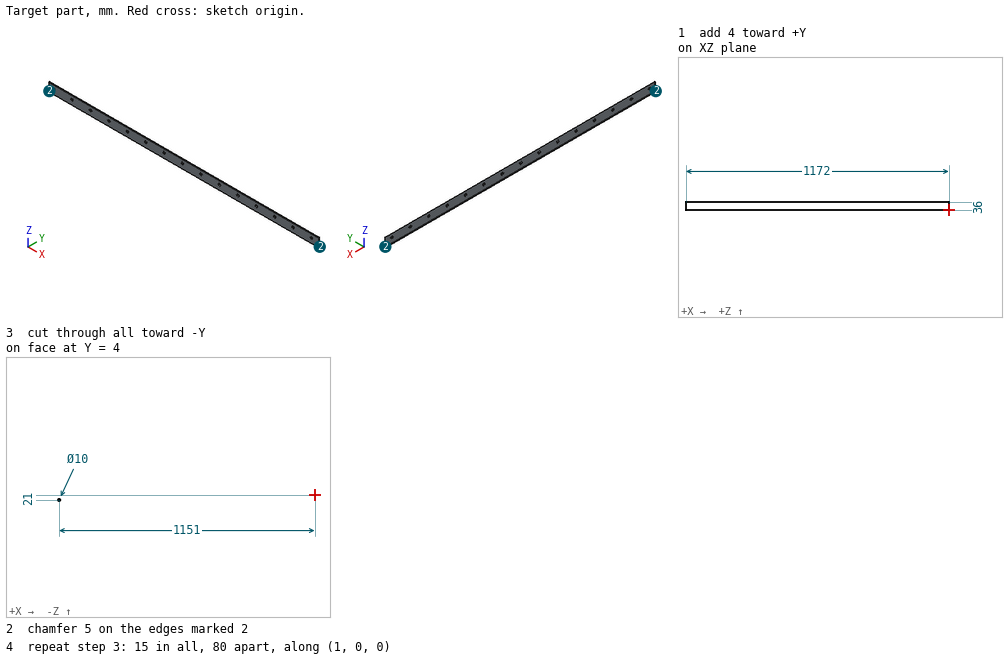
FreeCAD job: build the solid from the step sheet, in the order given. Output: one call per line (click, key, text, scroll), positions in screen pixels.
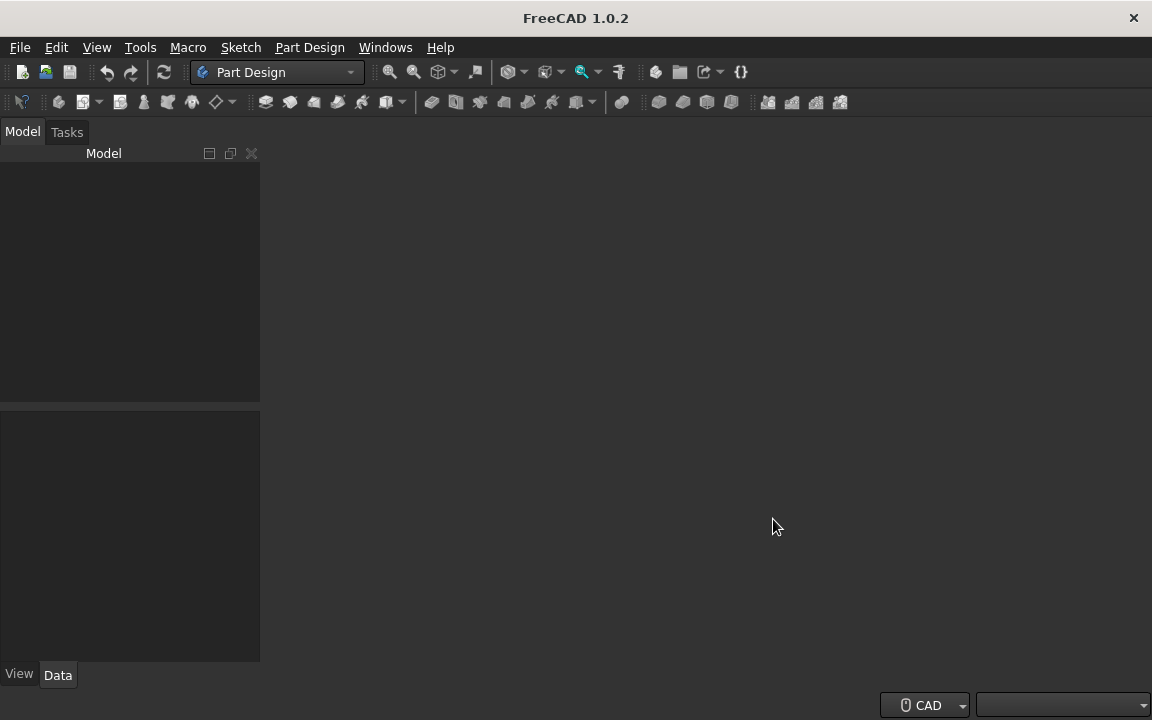
click(22, 72)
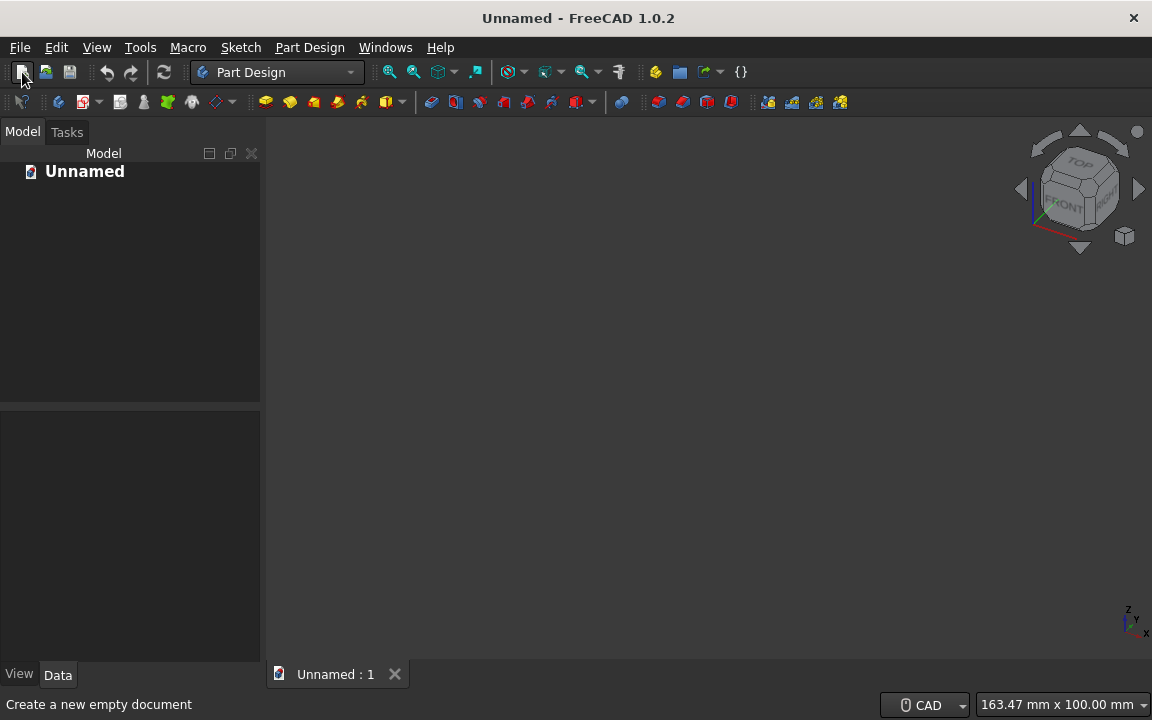
click(84, 102)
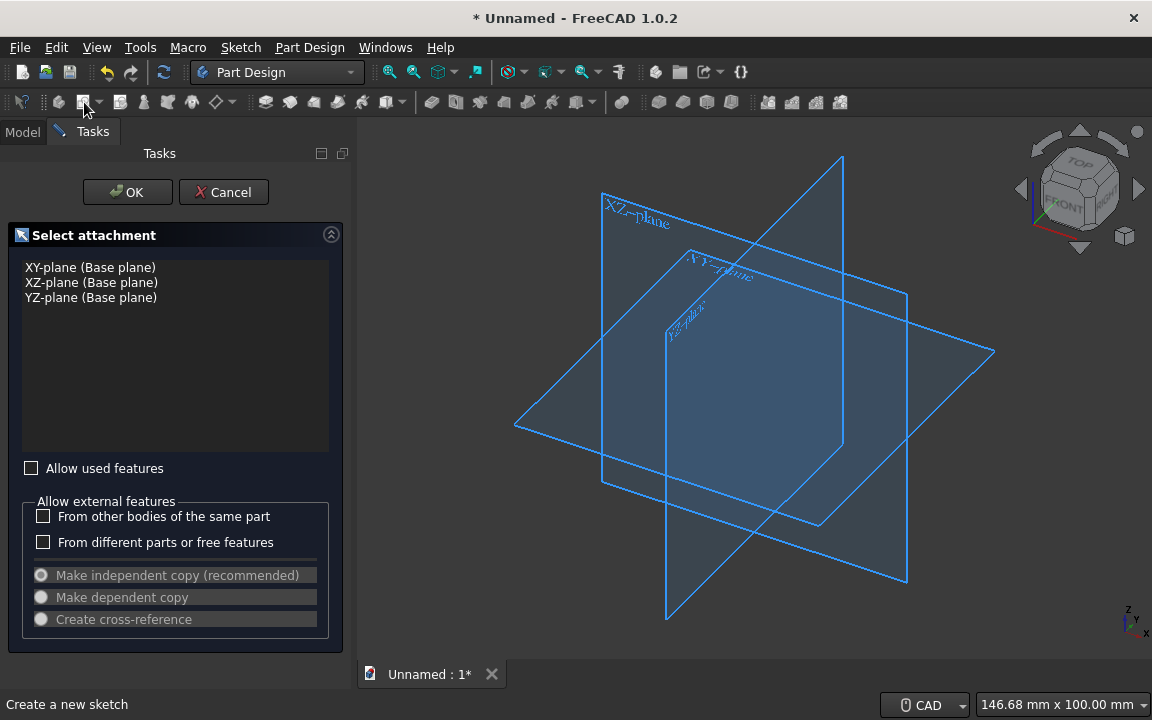
click(82, 282)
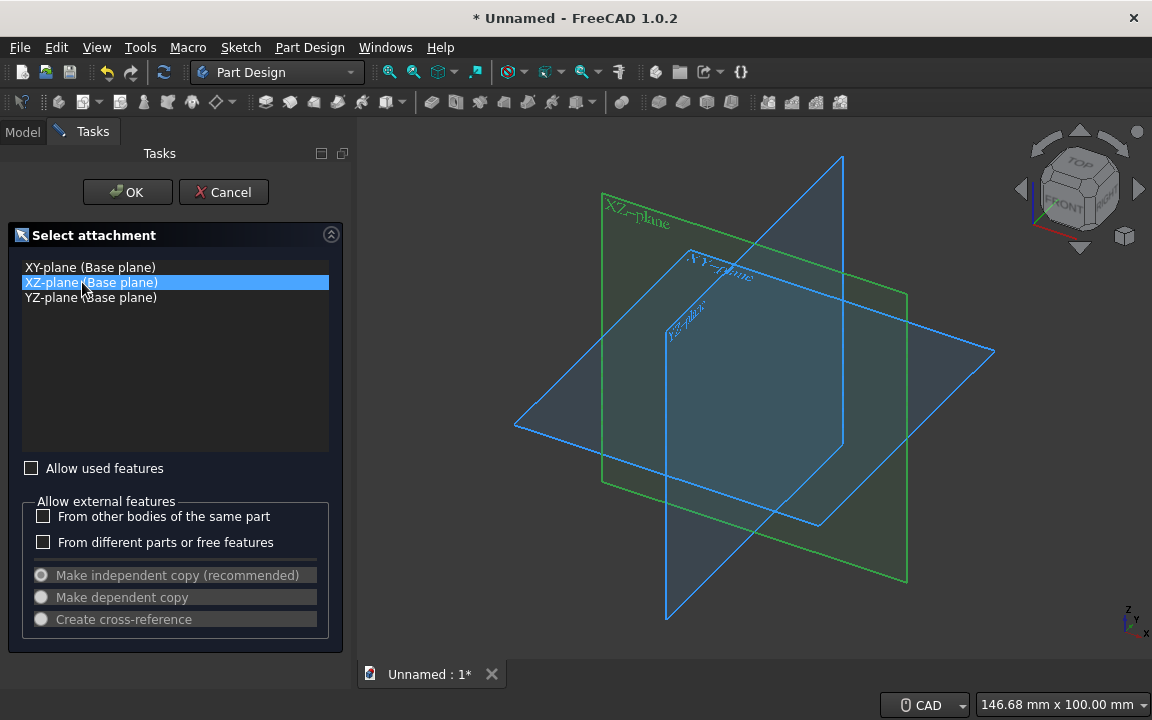
click(128, 192)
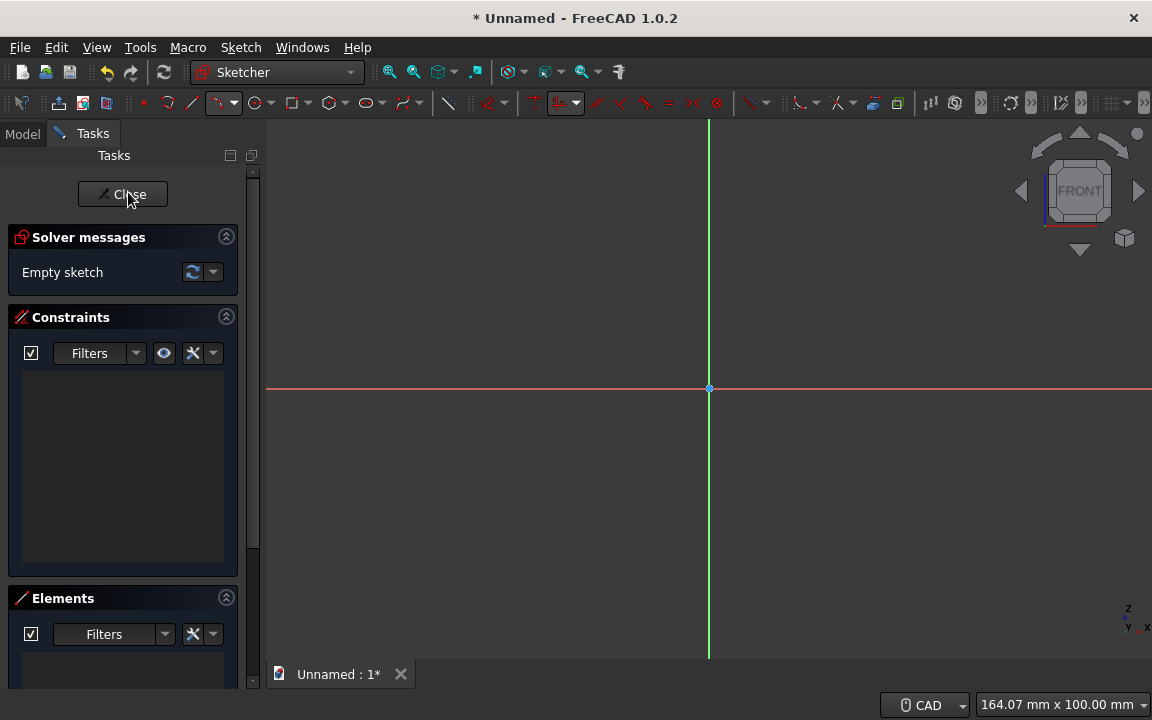
scroll(889, 397, down, 13)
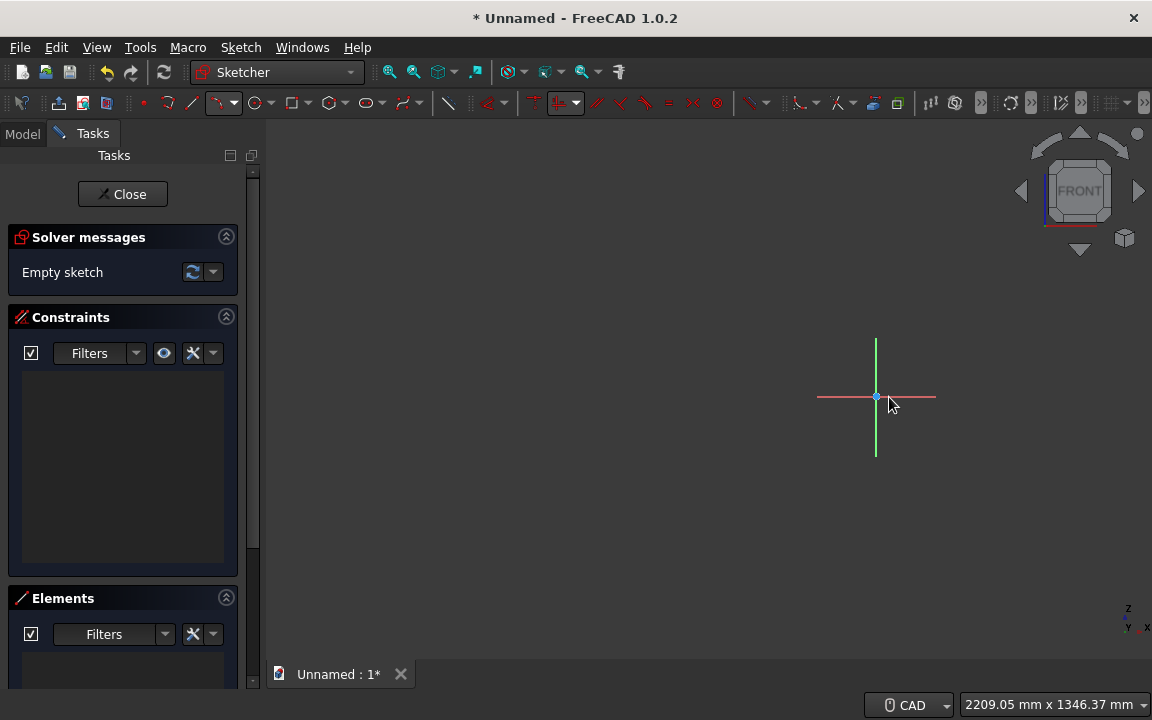
key(g)
key(r)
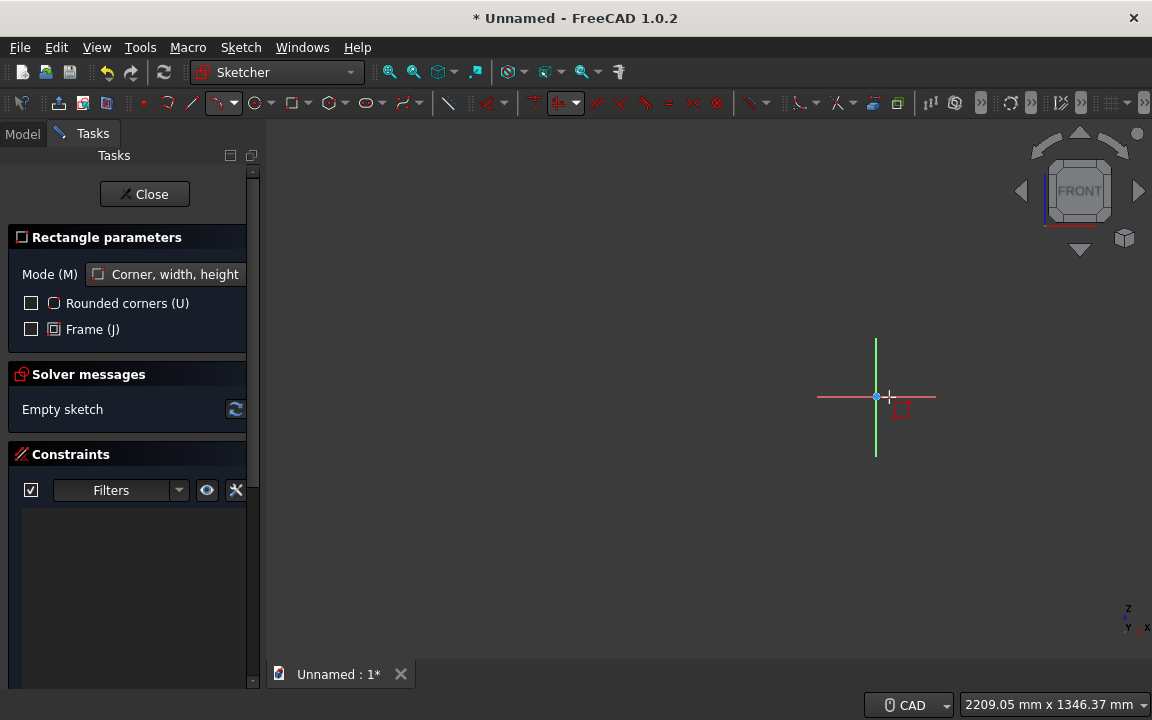
click(876, 397)
click(406, 382)
key(Escape)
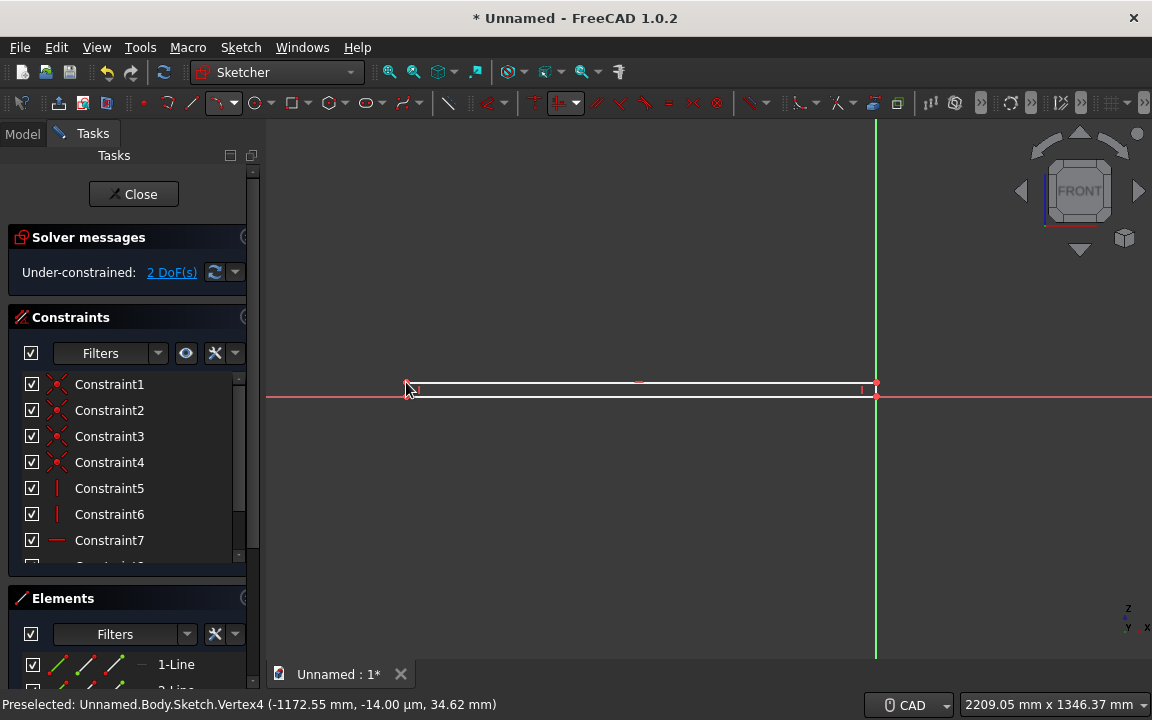
scroll(876, 390, up, 6)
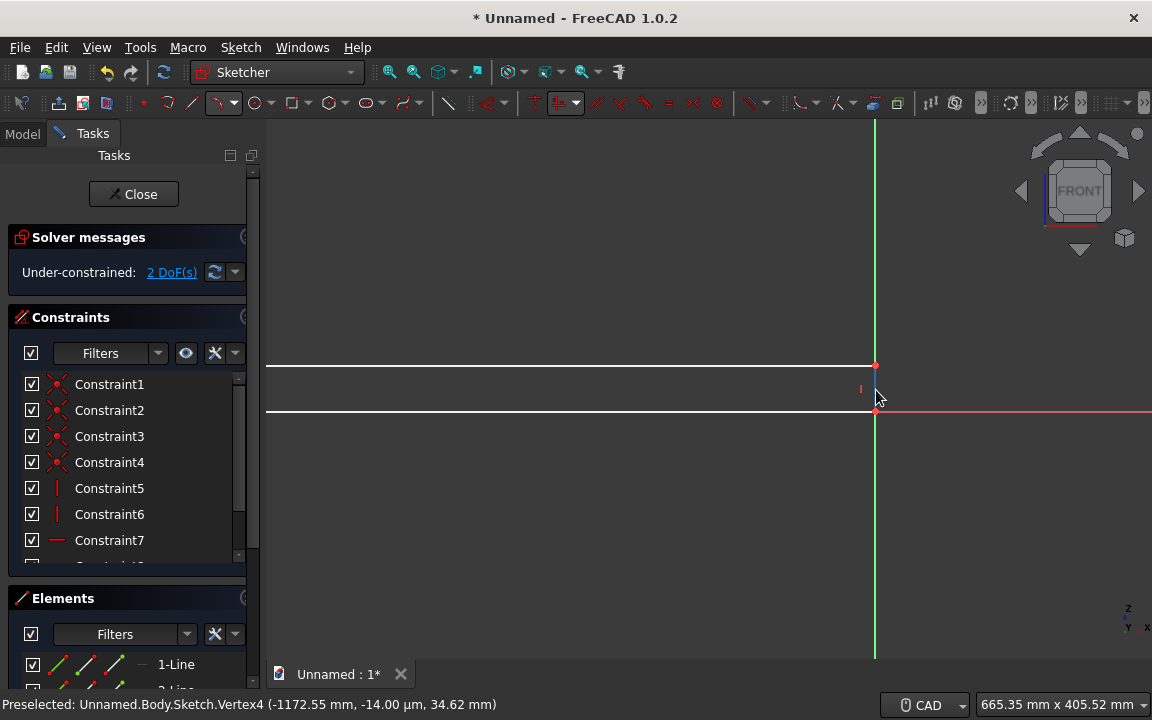
click(875, 389)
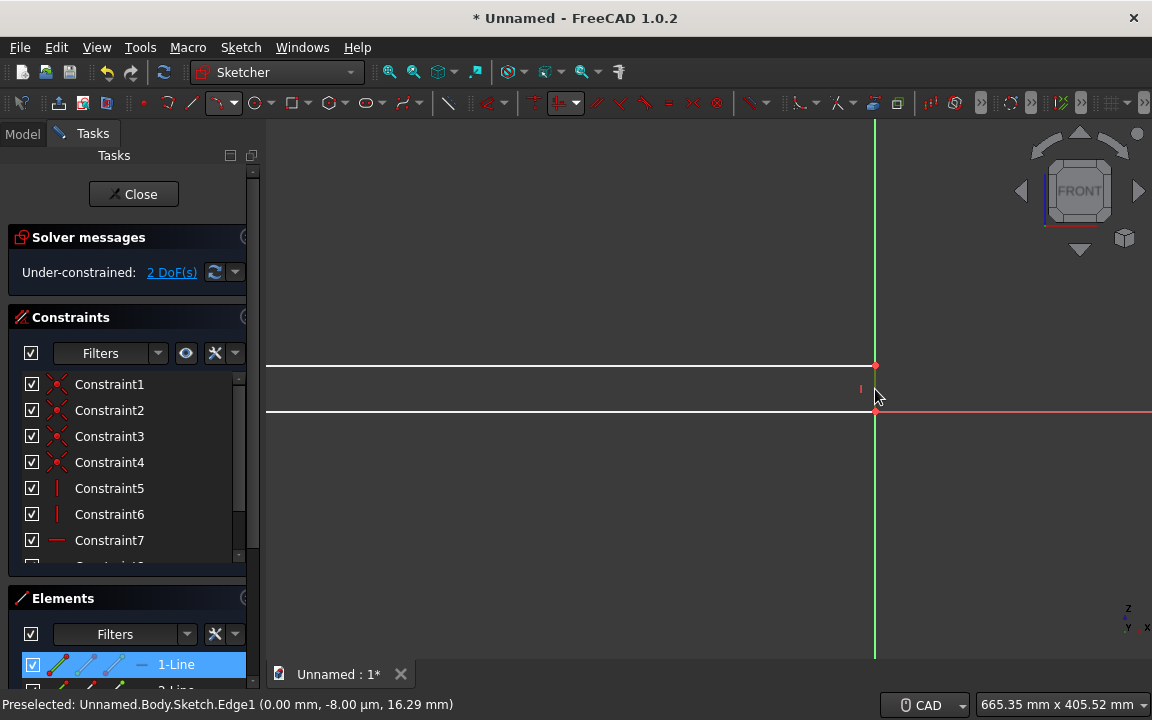
key(i)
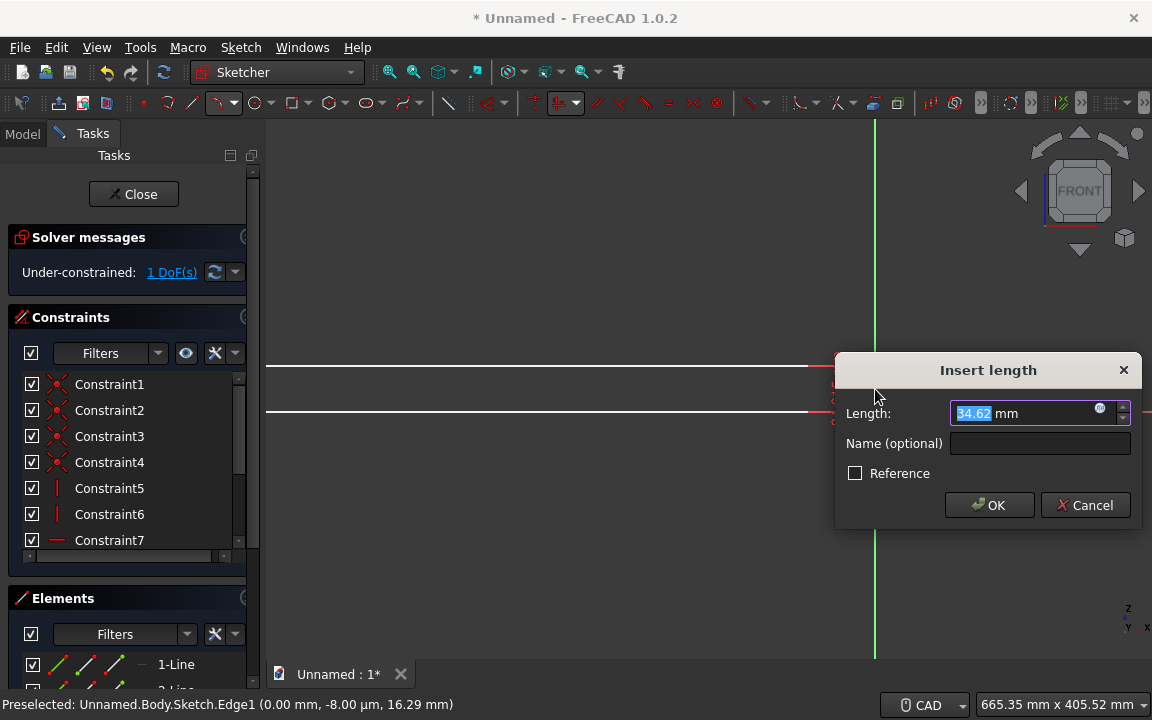
text(36)
key(Return)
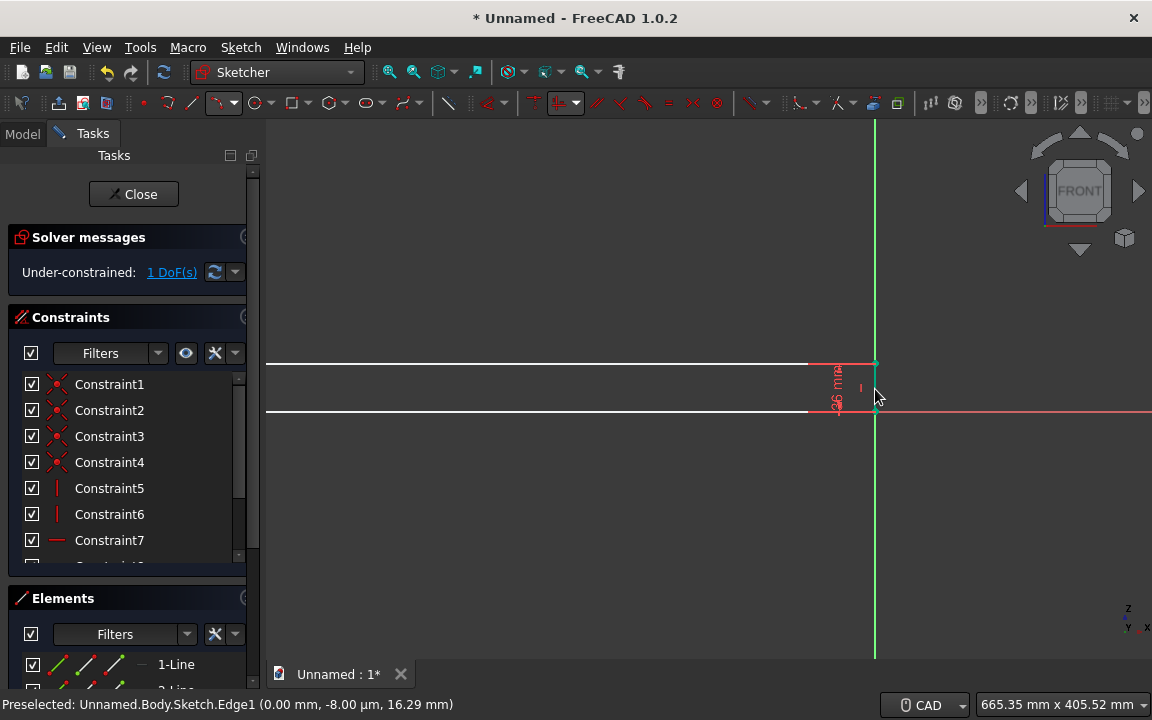
click(407, 364)